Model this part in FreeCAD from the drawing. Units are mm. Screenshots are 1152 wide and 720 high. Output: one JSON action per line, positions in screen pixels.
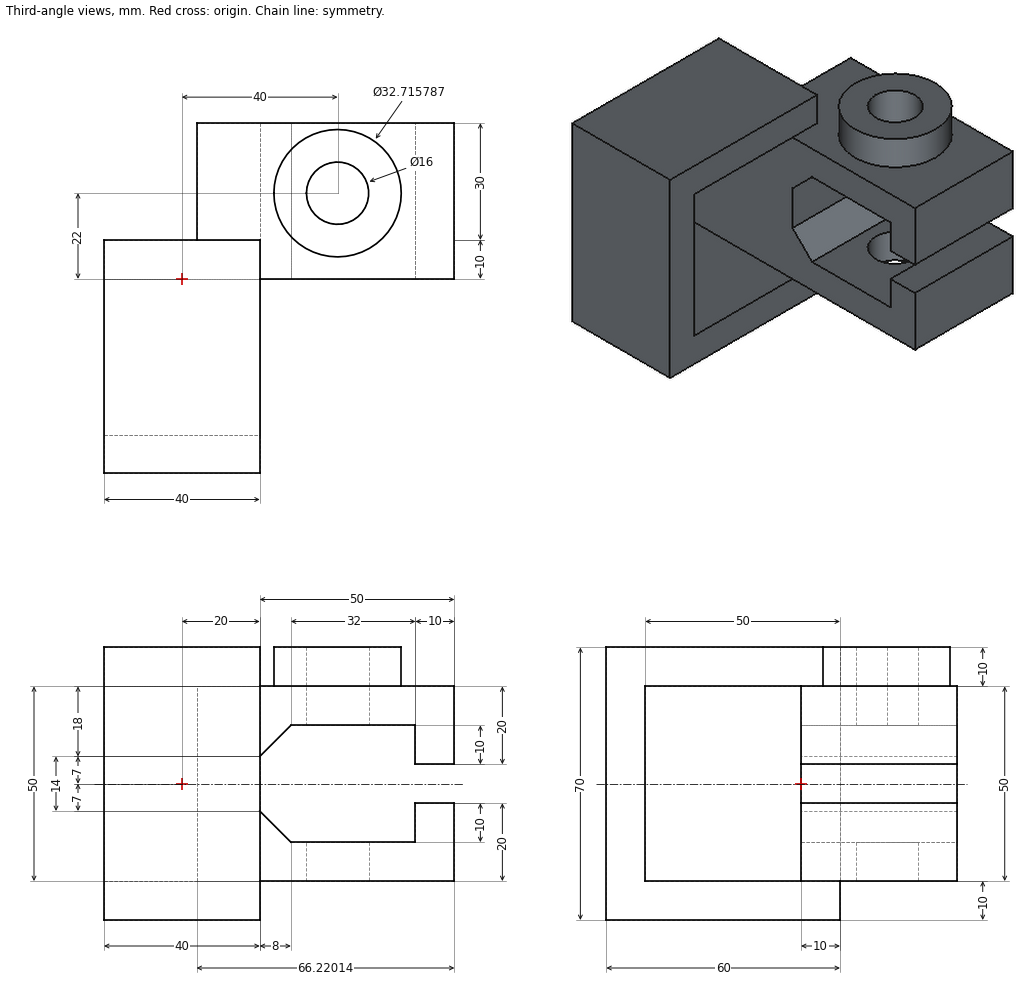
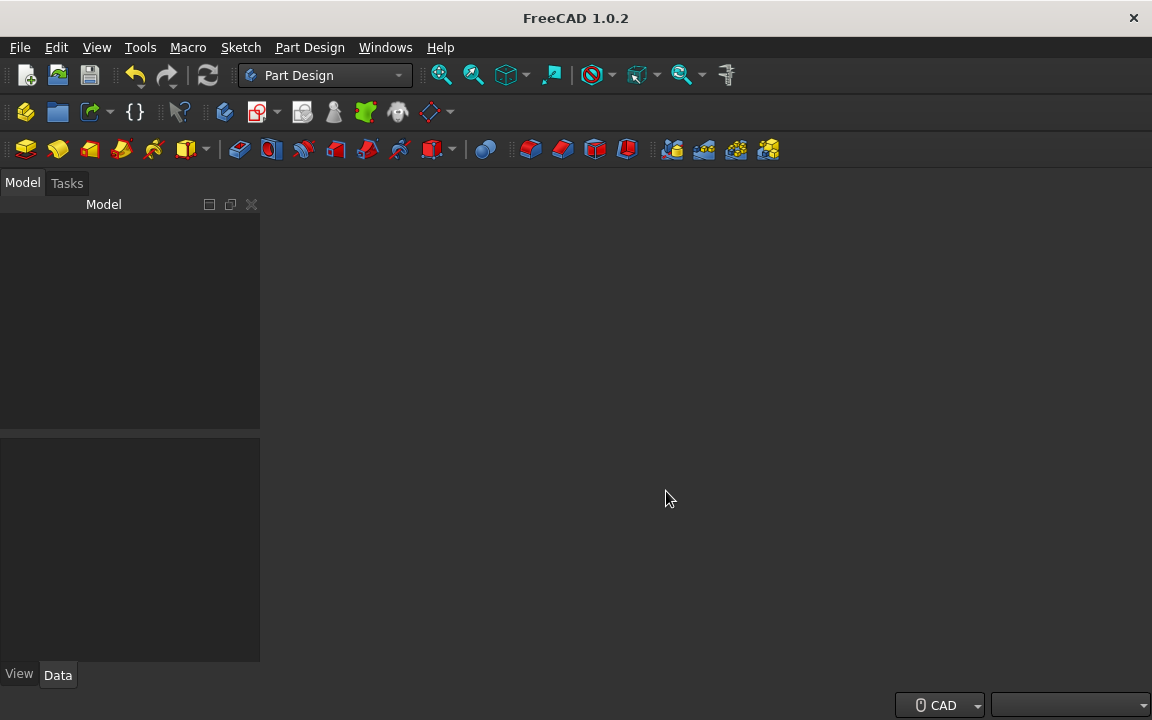
{"action": "left_click", "coordinate": [26, 76]}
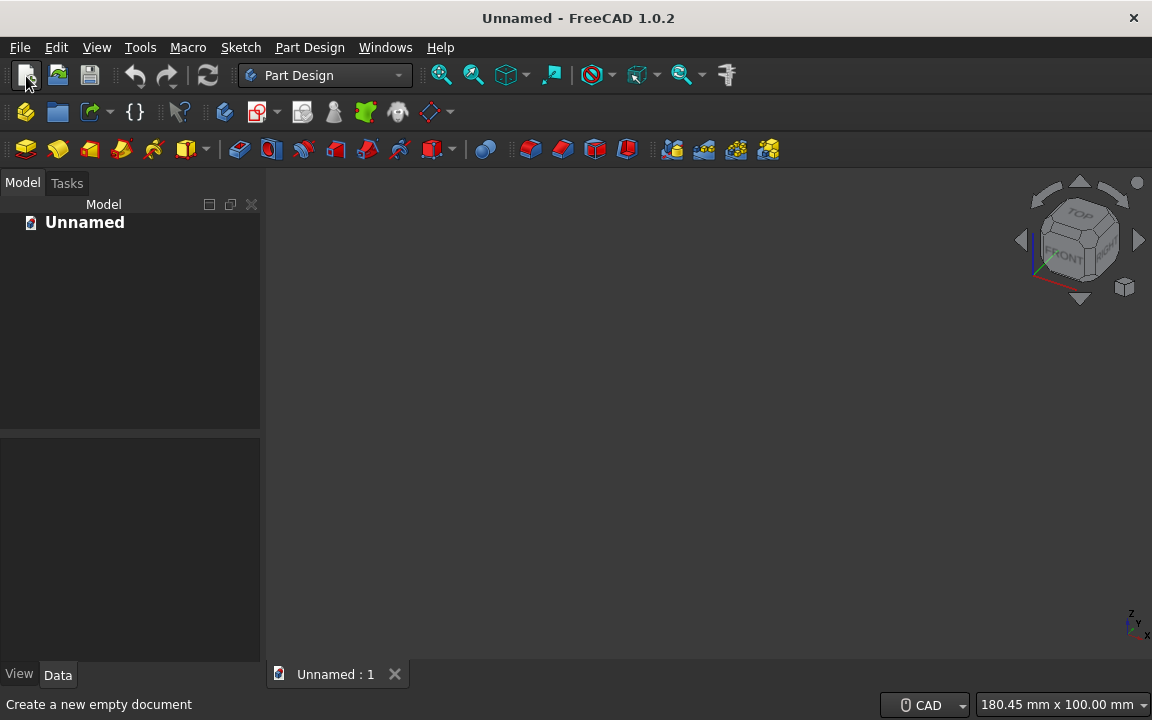
{"action": "left_click", "coordinate": [258, 112]}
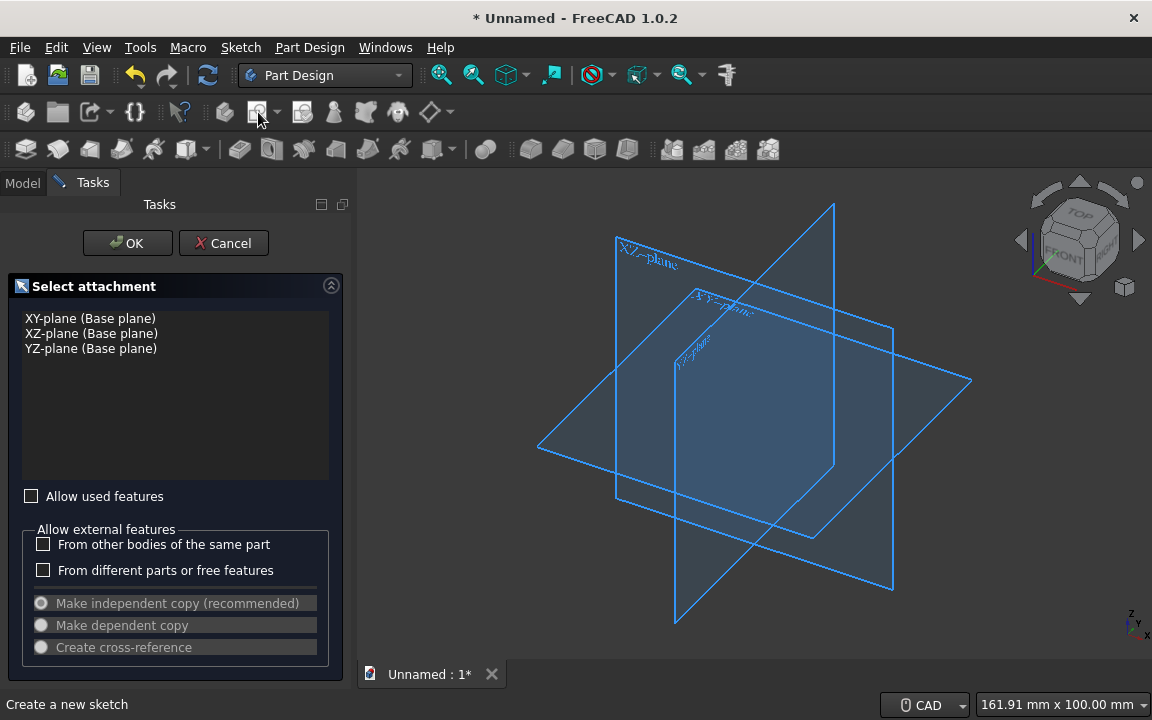
{"action": "left_click", "coordinate": [82, 334]}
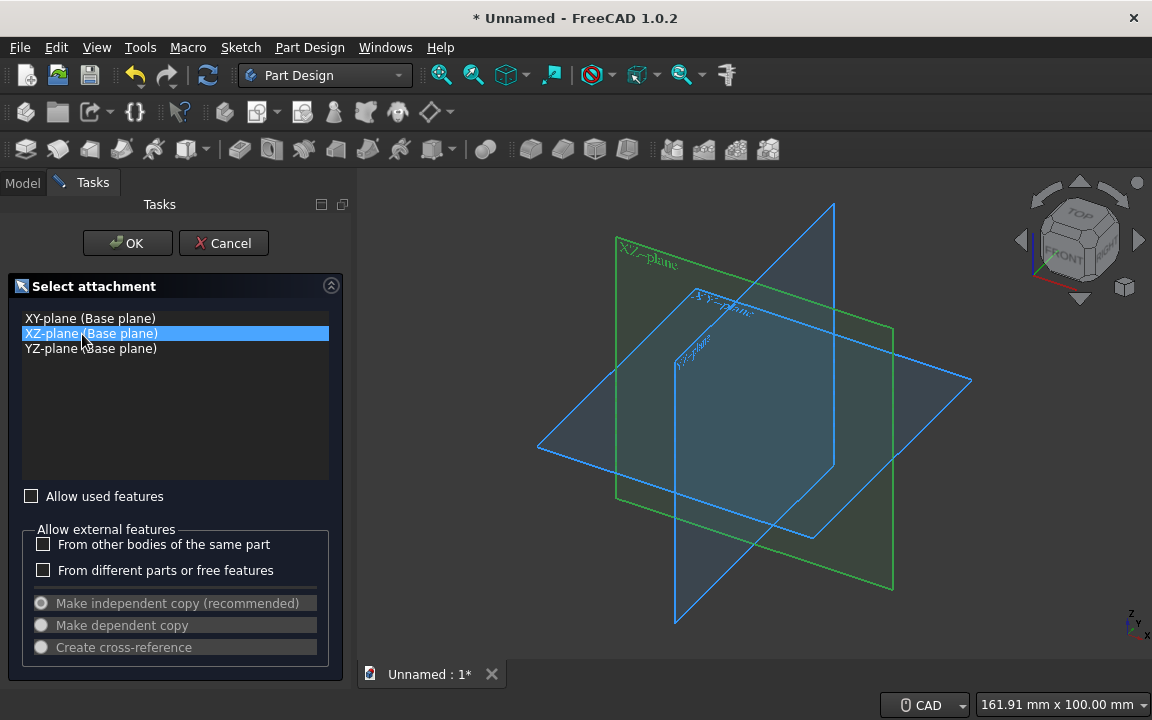
{"action": "left_click", "coordinate": [128, 243]}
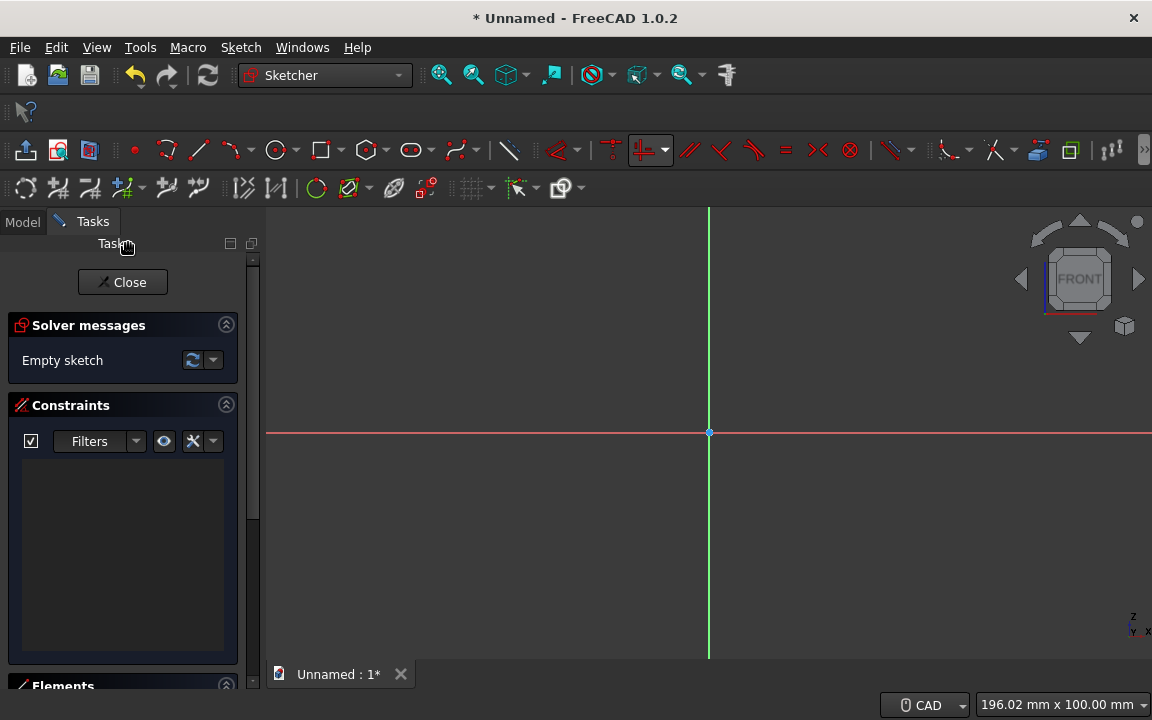
{"action": "key", "text": "g v"}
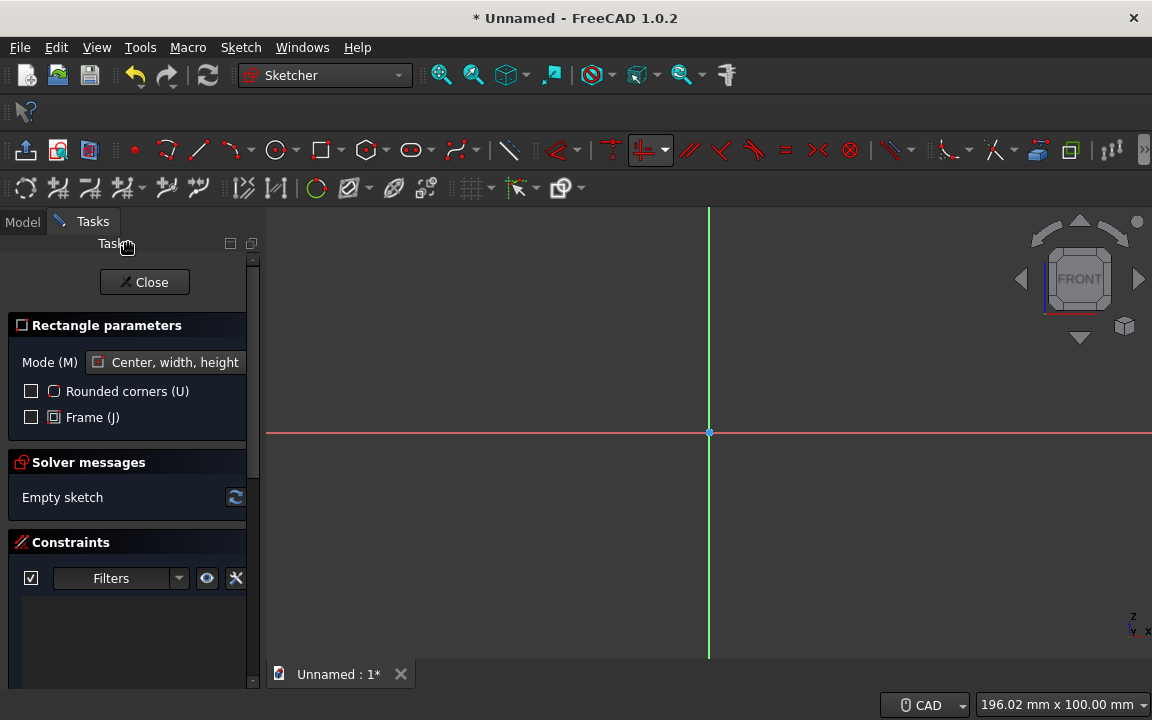
{"action": "left_click", "coordinate": [709, 433]}
{"action": "left_click", "coordinate": [799, 320]}
{"action": "key", "text": "Escape"}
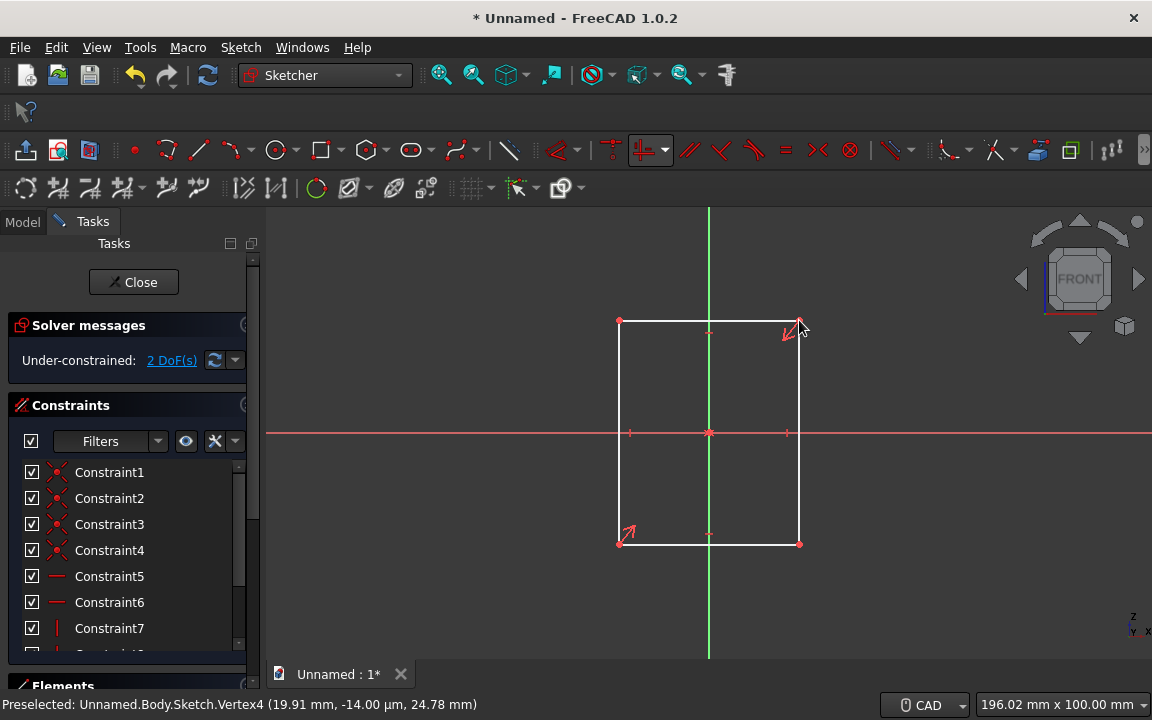
{"action": "key", "text": "d"}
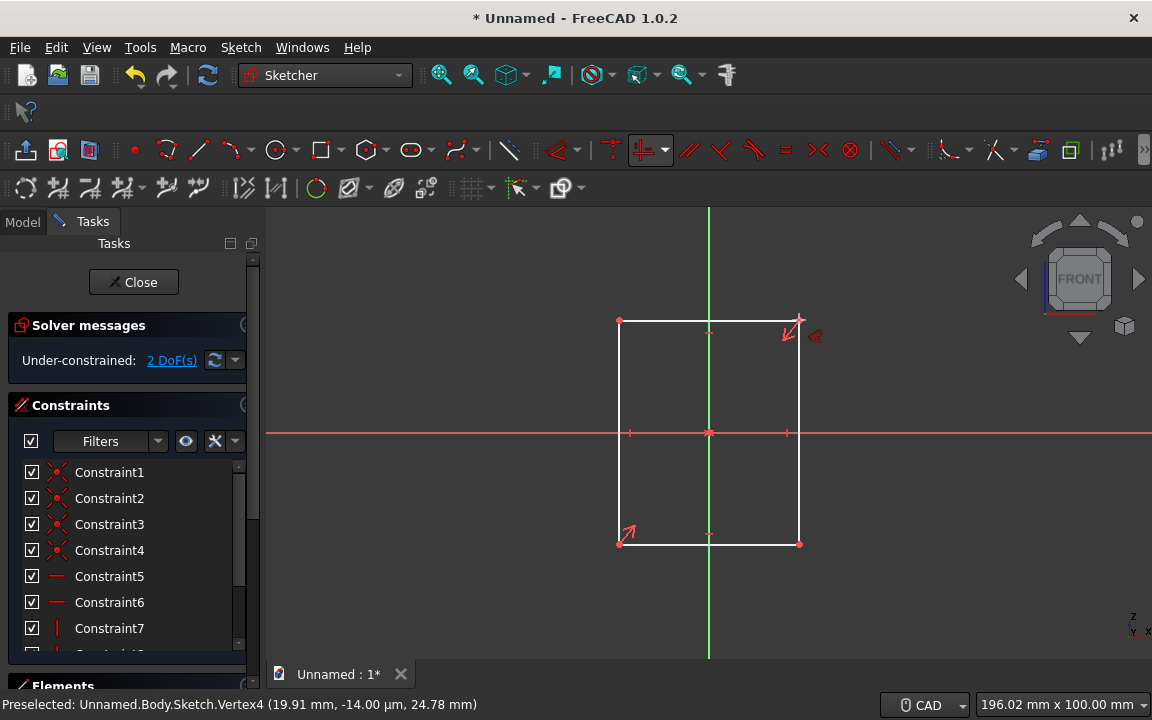
{"action": "left_click", "coordinate": [673, 545]}
{"action": "left_click", "coordinate": [668, 579]}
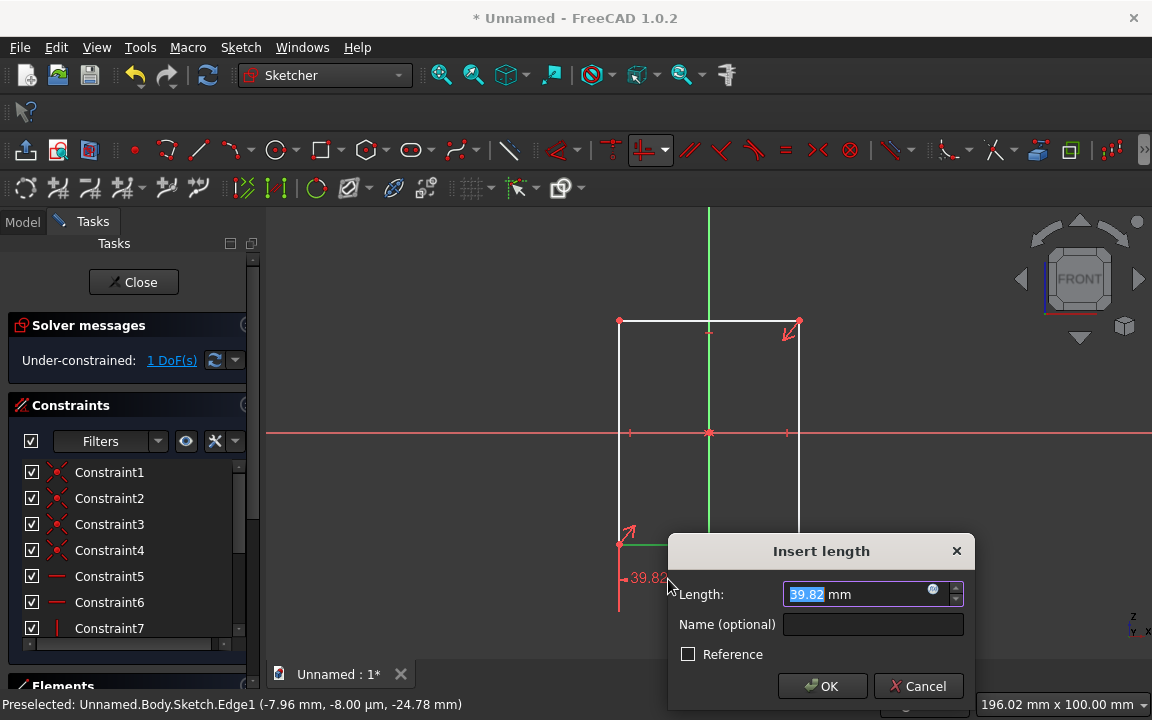
{"action": "type", "text": "40"}
{"action": "key", "text": "Return"}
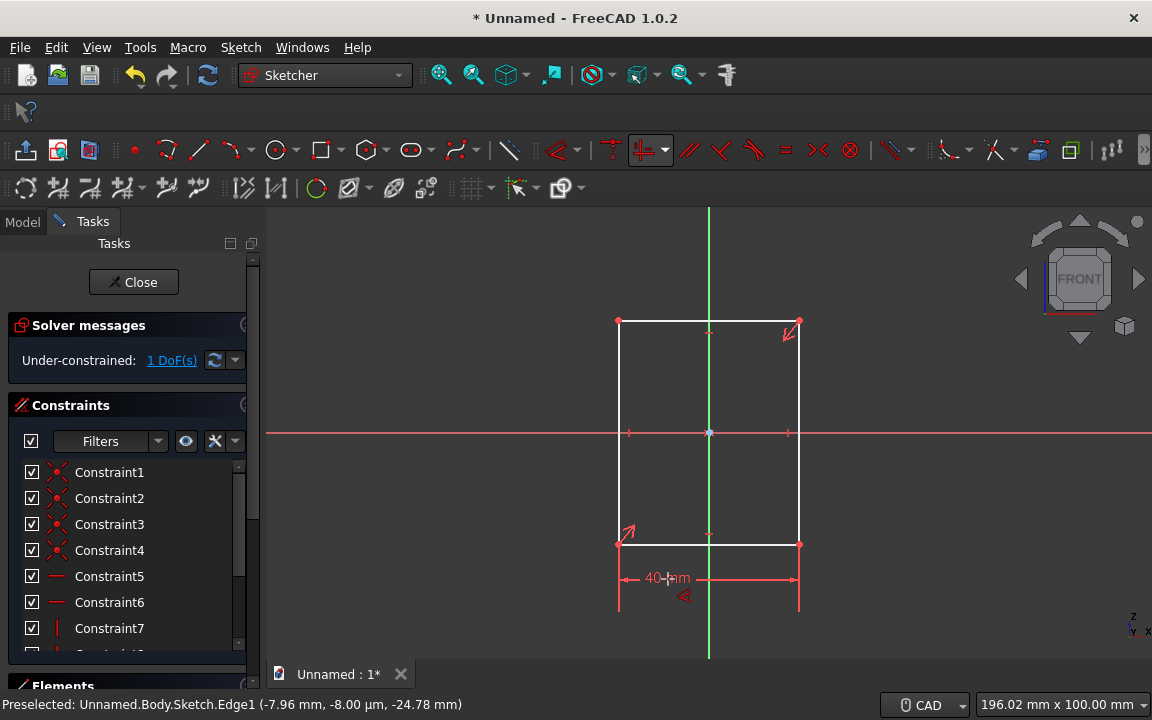
{"action": "left_click", "coordinate": [799, 478]}
{"action": "left_click", "coordinate": [833, 381]}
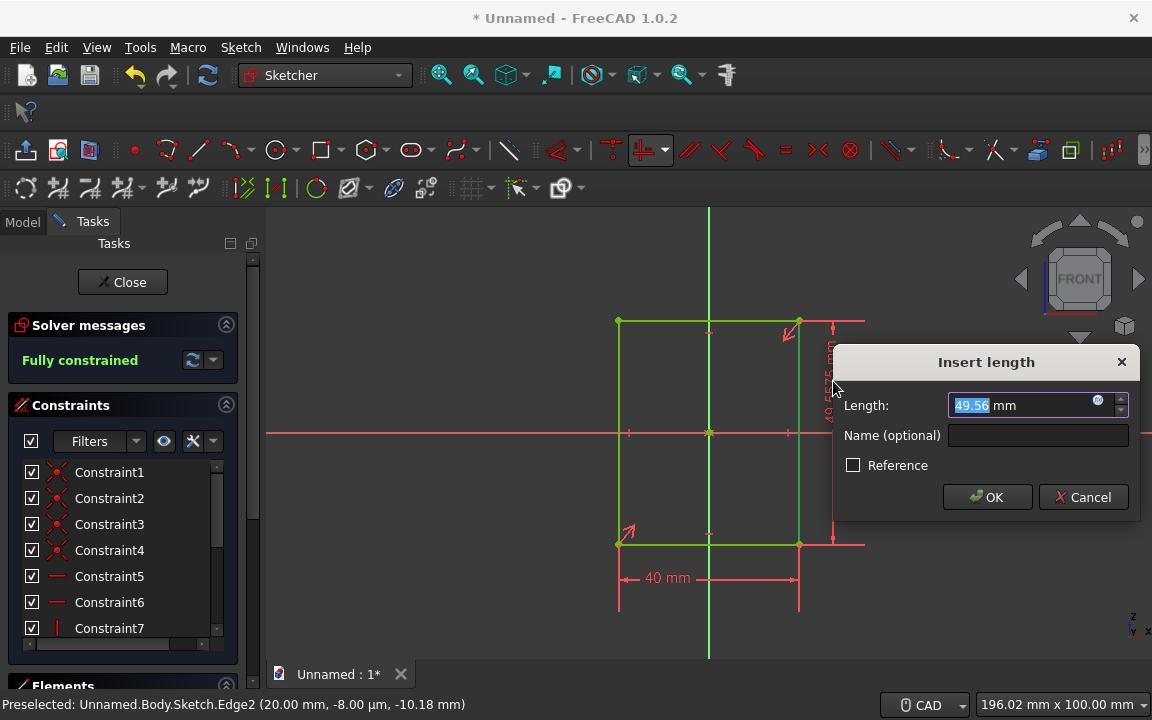
{"action": "type", "text": "50"}
{"action": "key", "text": "Return"}
{"action": "key", "text": "Escape"}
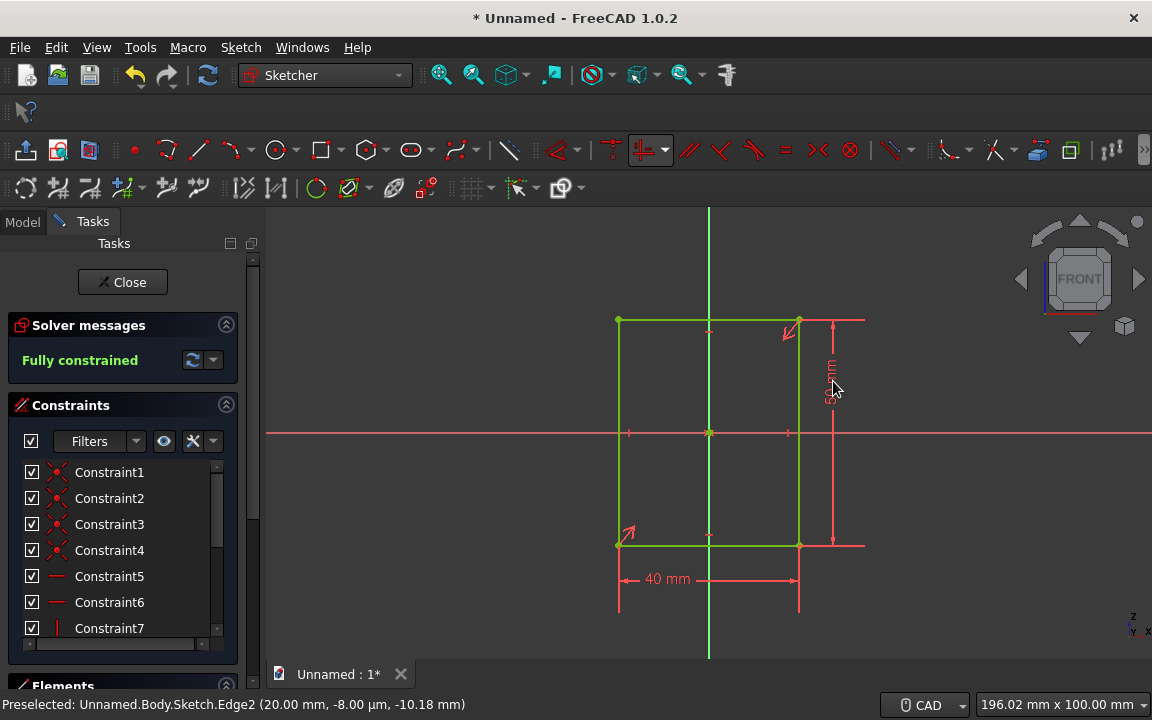
{"action": "left_click", "coordinate": [123, 282]}